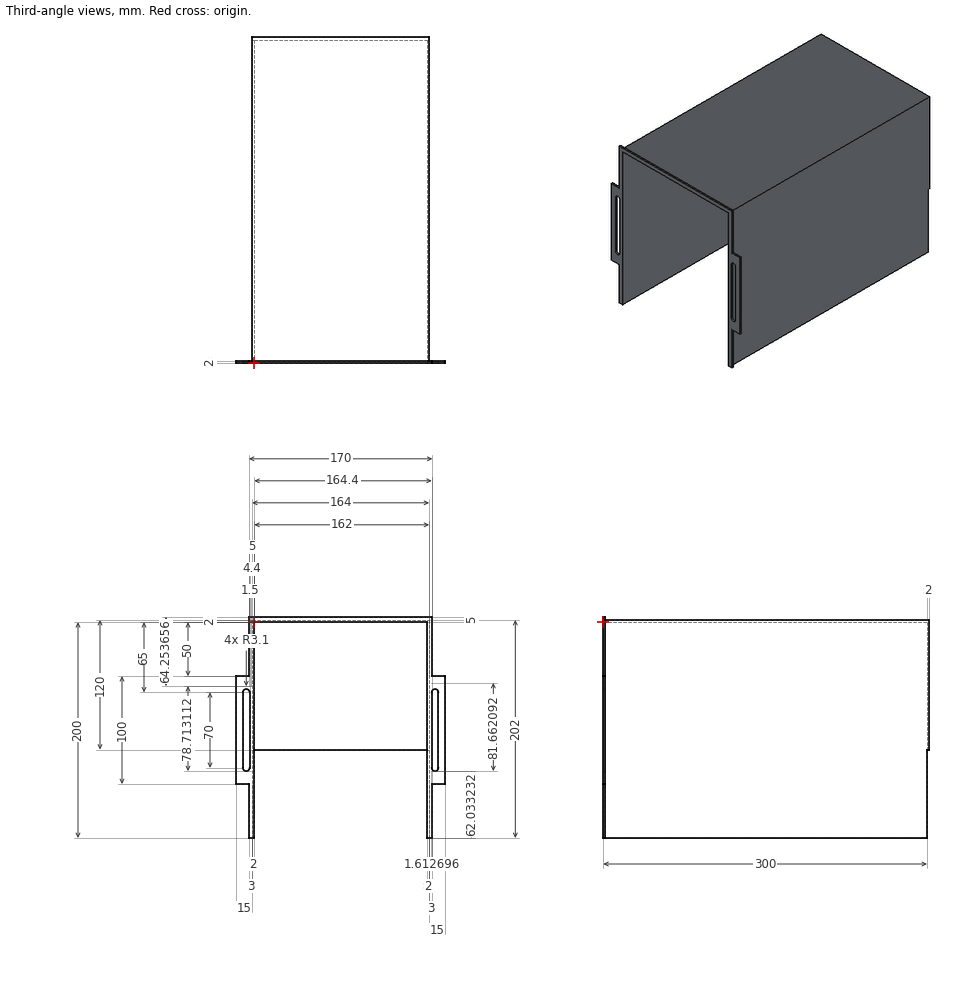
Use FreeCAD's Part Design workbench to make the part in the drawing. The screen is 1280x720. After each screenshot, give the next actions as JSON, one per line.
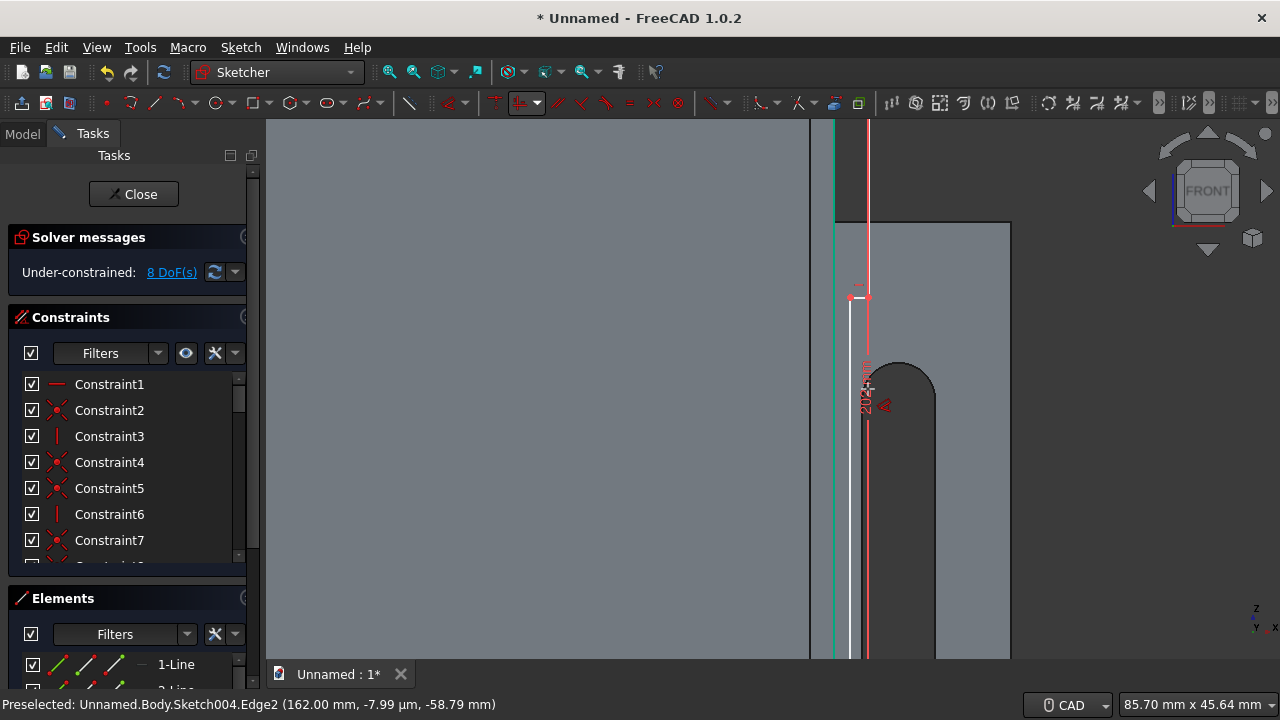
{"action": "scroll", "coordinate": [836, 327], "scroll_direction": "down", "scroll_amount": 10}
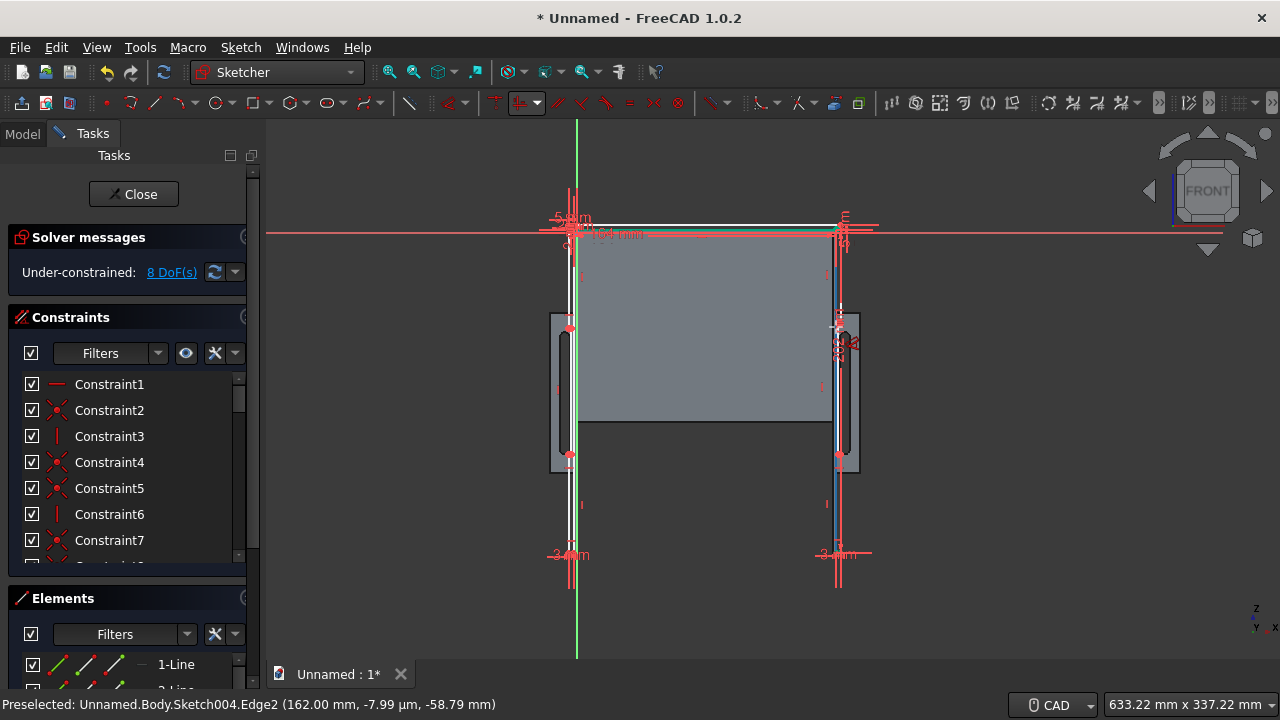
{"action": "scroll", "coordinate": [759, 225], "scroll_direction": "up", "scroll_amount": 6}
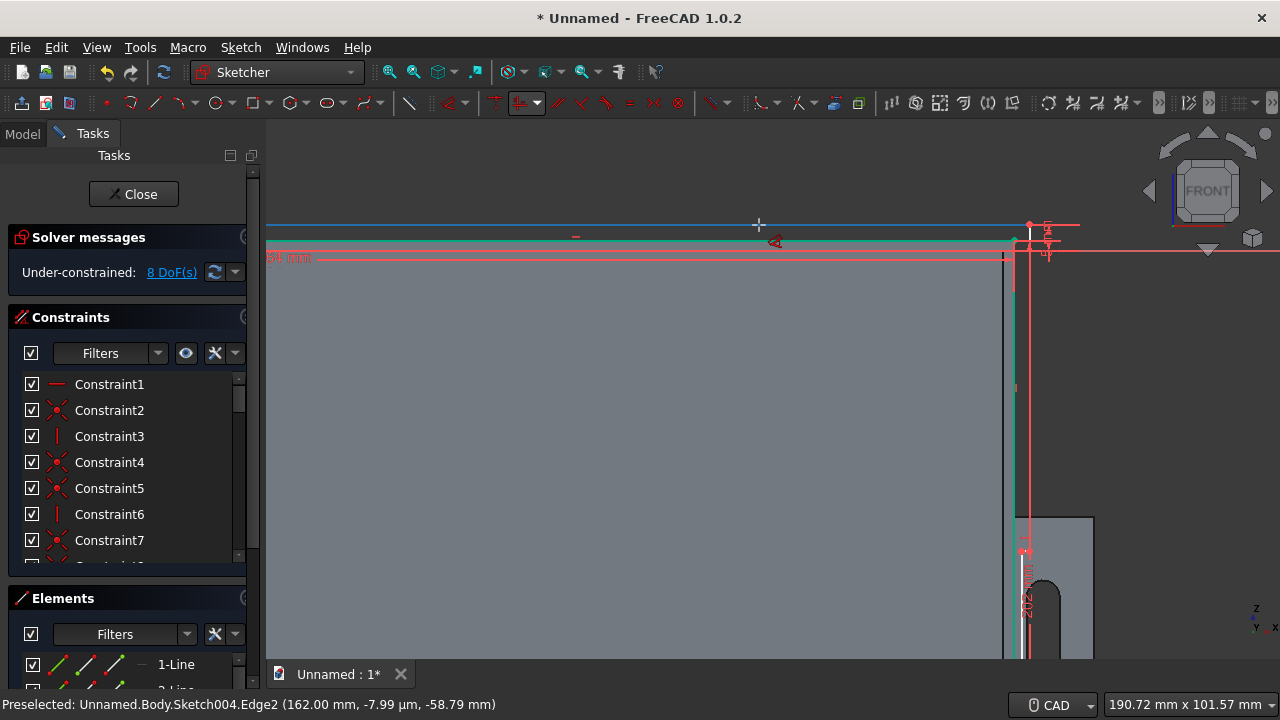
{"action": "left_click", "coordinate": [759, 225]}
{"action": "left_click", "coordinate": [662, 191]}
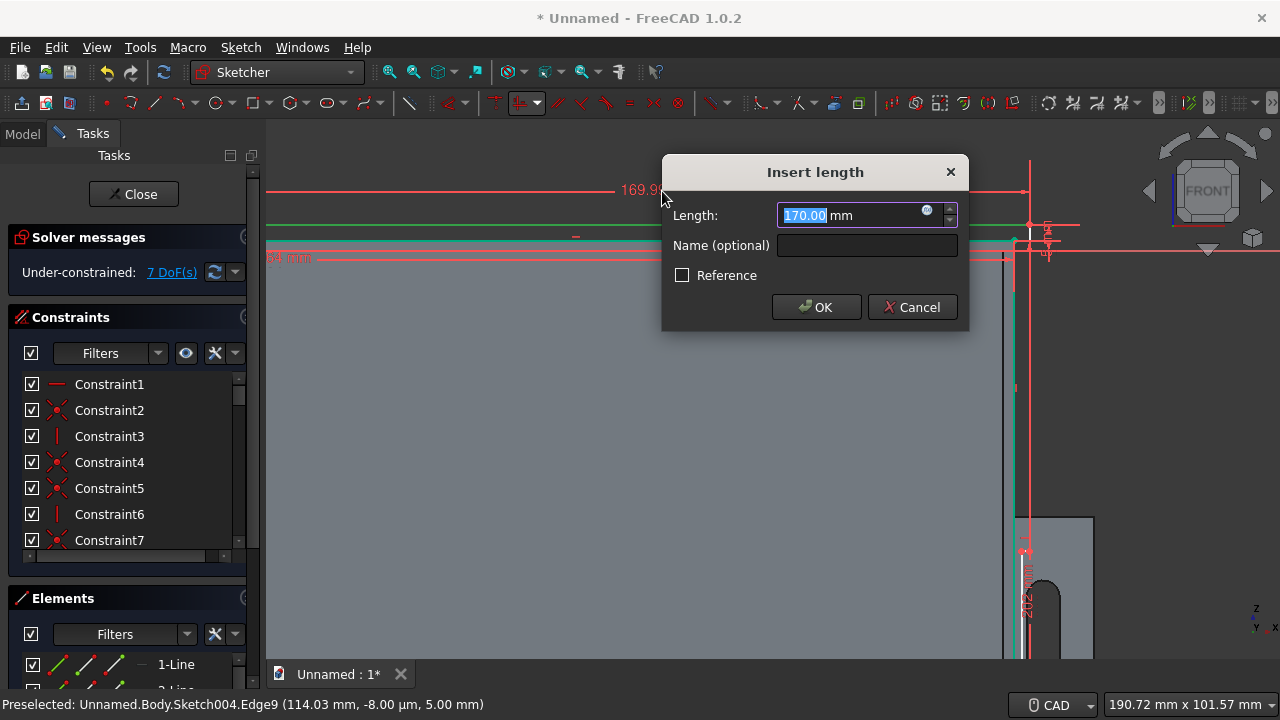
{"action": "type", "text": "170"}
{"action": "key", "text": "Return"}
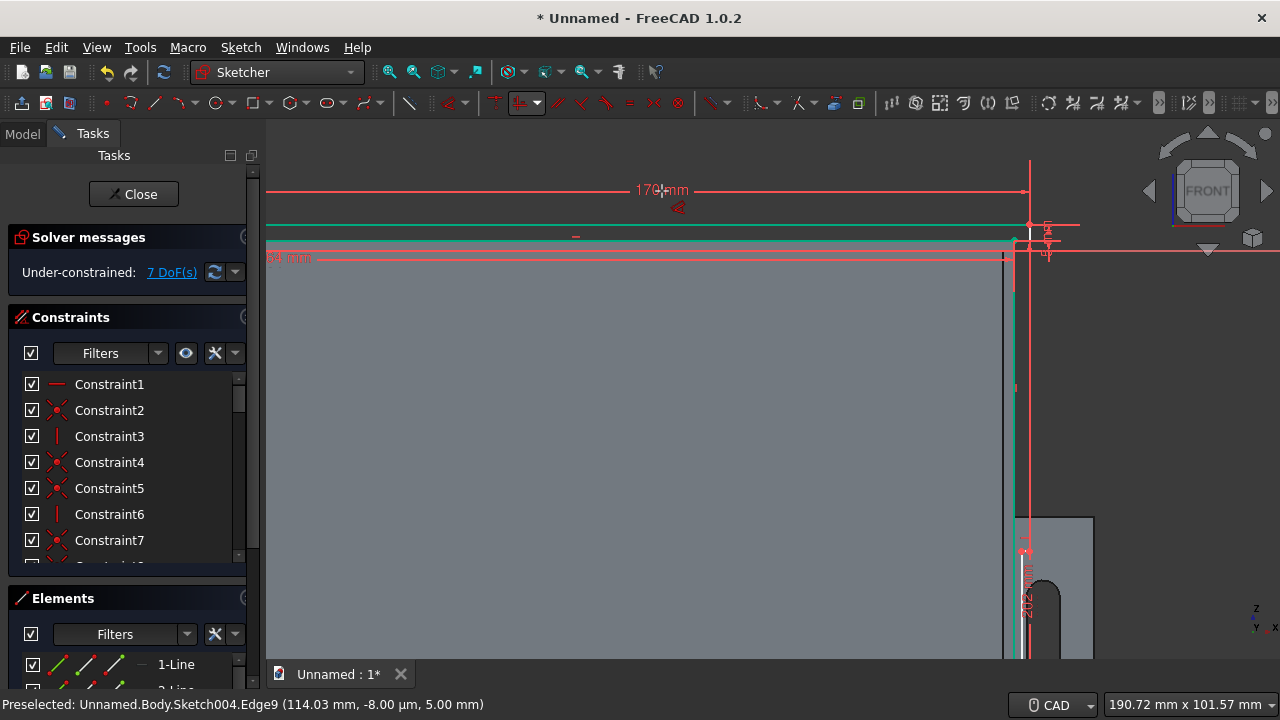
{"action": "scroll", "coordinate": [759, 225], "scroll_direction": "down", "scroll_amount": 6}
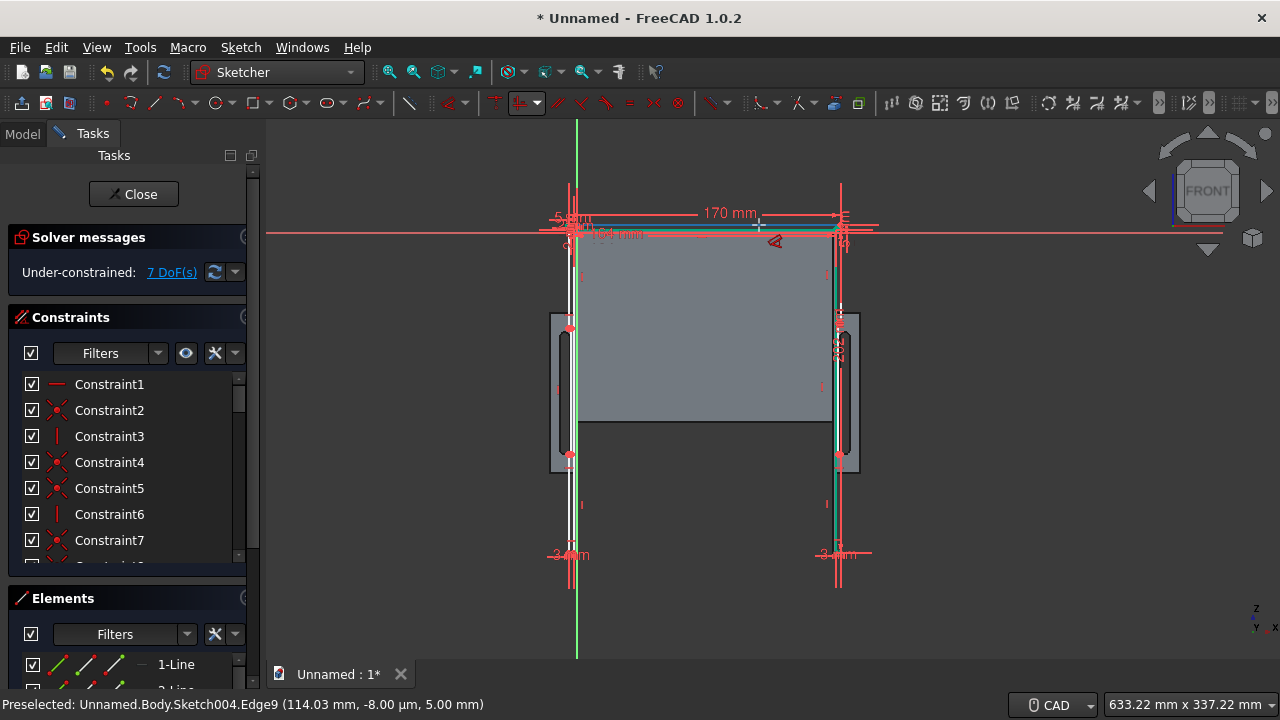
{"action": "scroll", "coordinate": [570, 328], "scroll_direction": "up", "scroll_amount": 15}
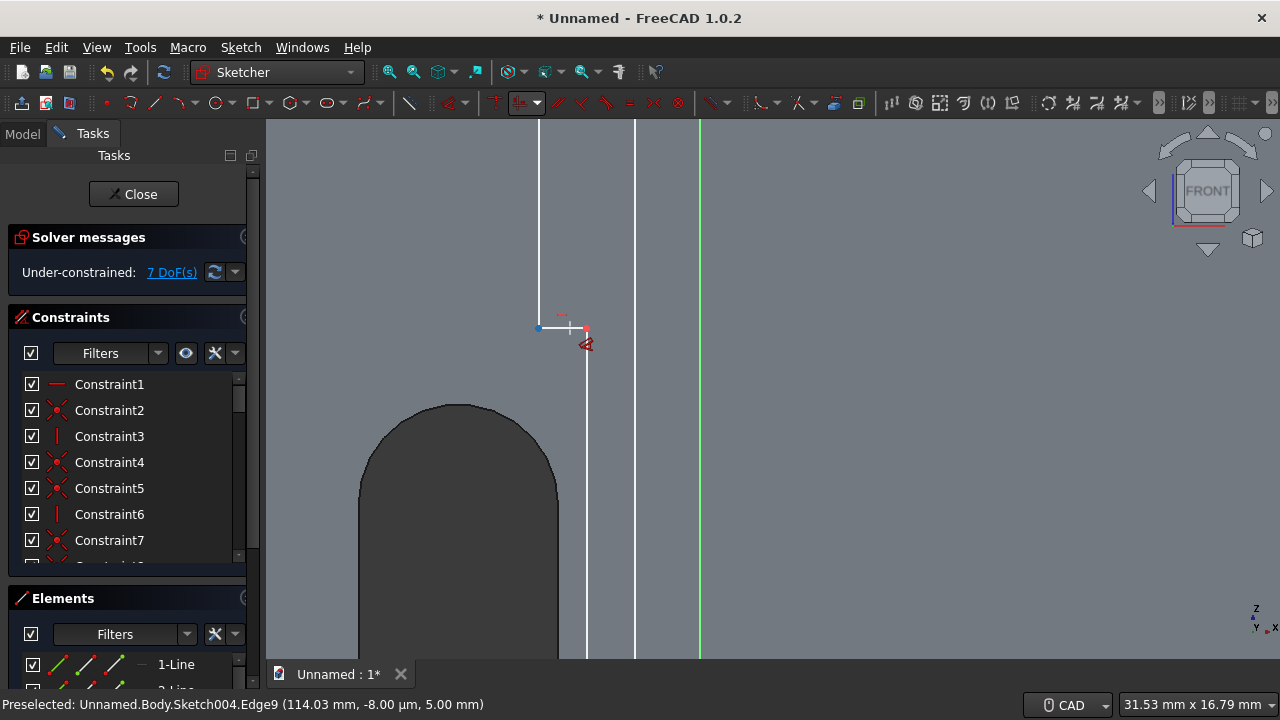
{"action": "left_click", "coordinate": [563, 328]}
{"action": "left_click", "coordinate": [563, 294]}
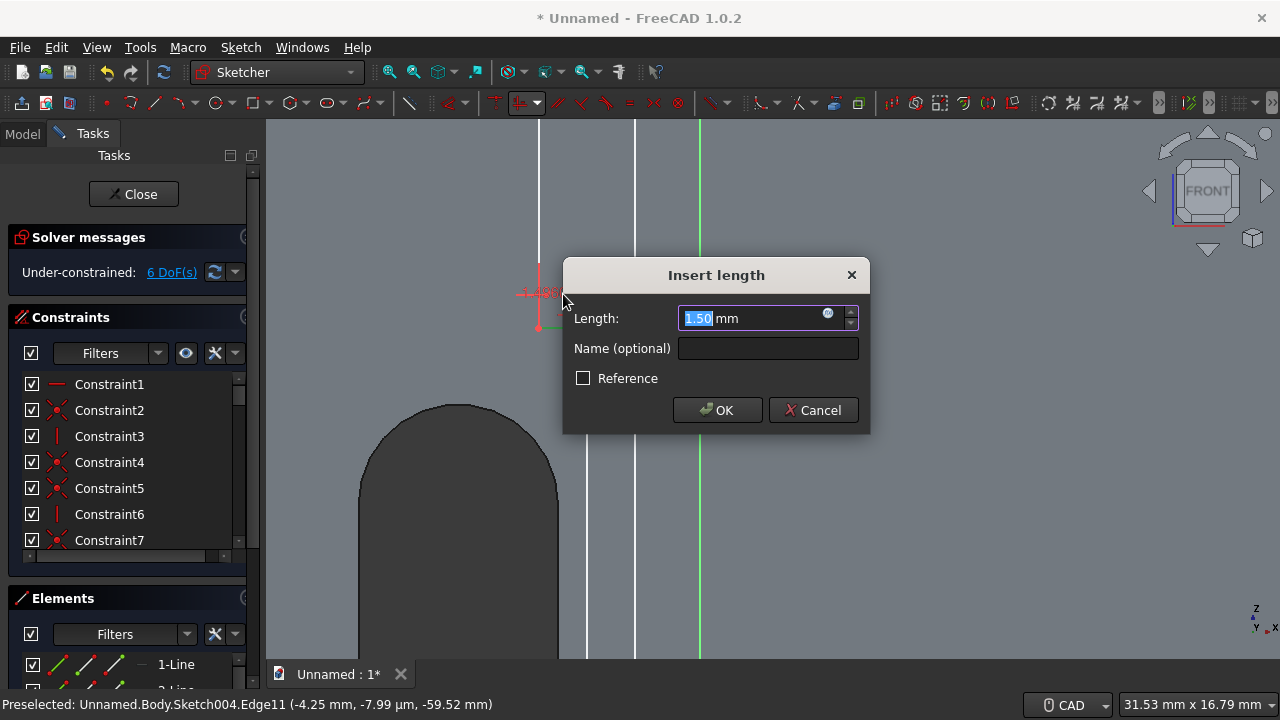
{"action": "type", "text": "1.5"}
{"action": "key", "text": "Return"}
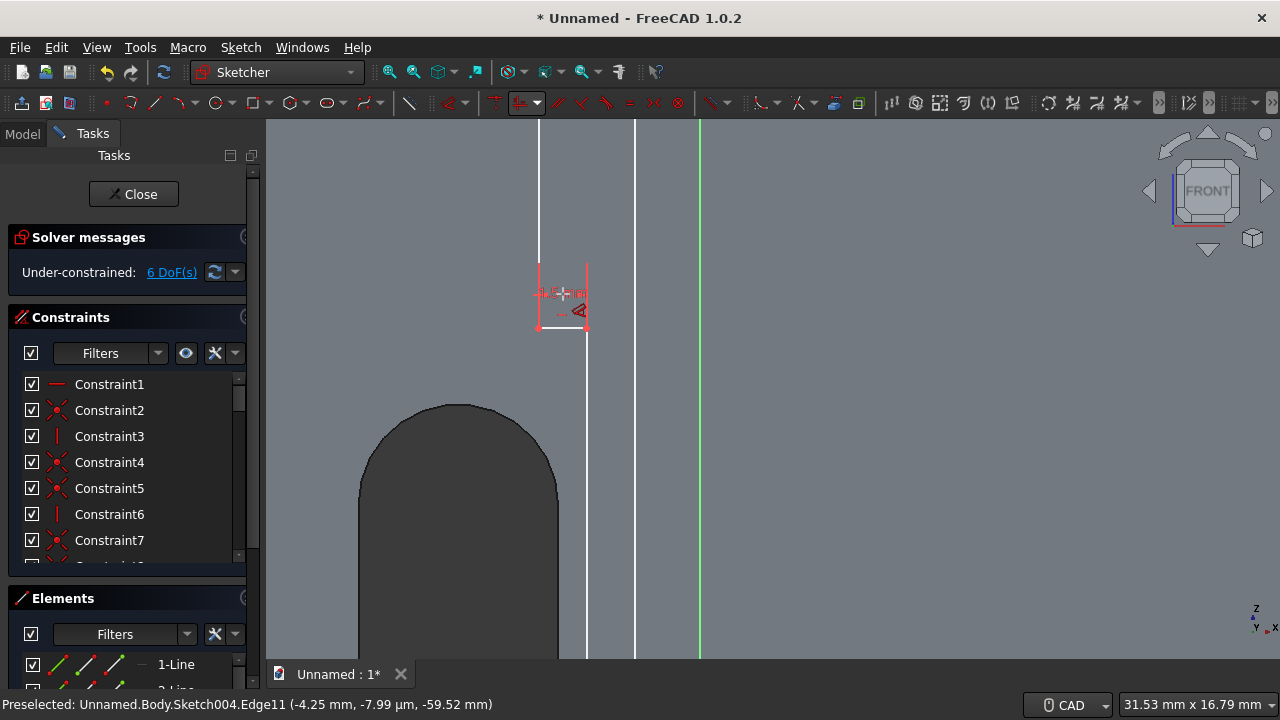
{"action": "scroll", "coordinate": [570, 328], "scroll_direction": "down", "scroll_amount": 15}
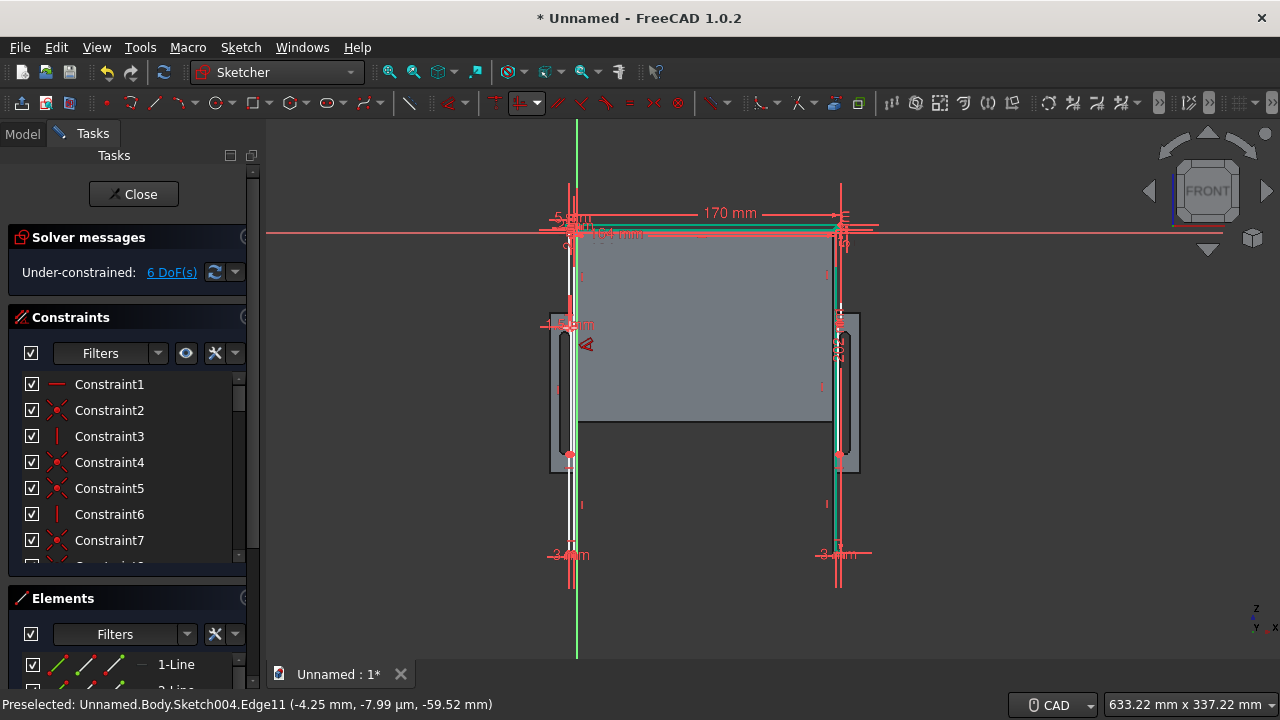
{"action": "scroll", "coordinate": [574, 327], "scroll_direction": "up", "scroll_amount": 9}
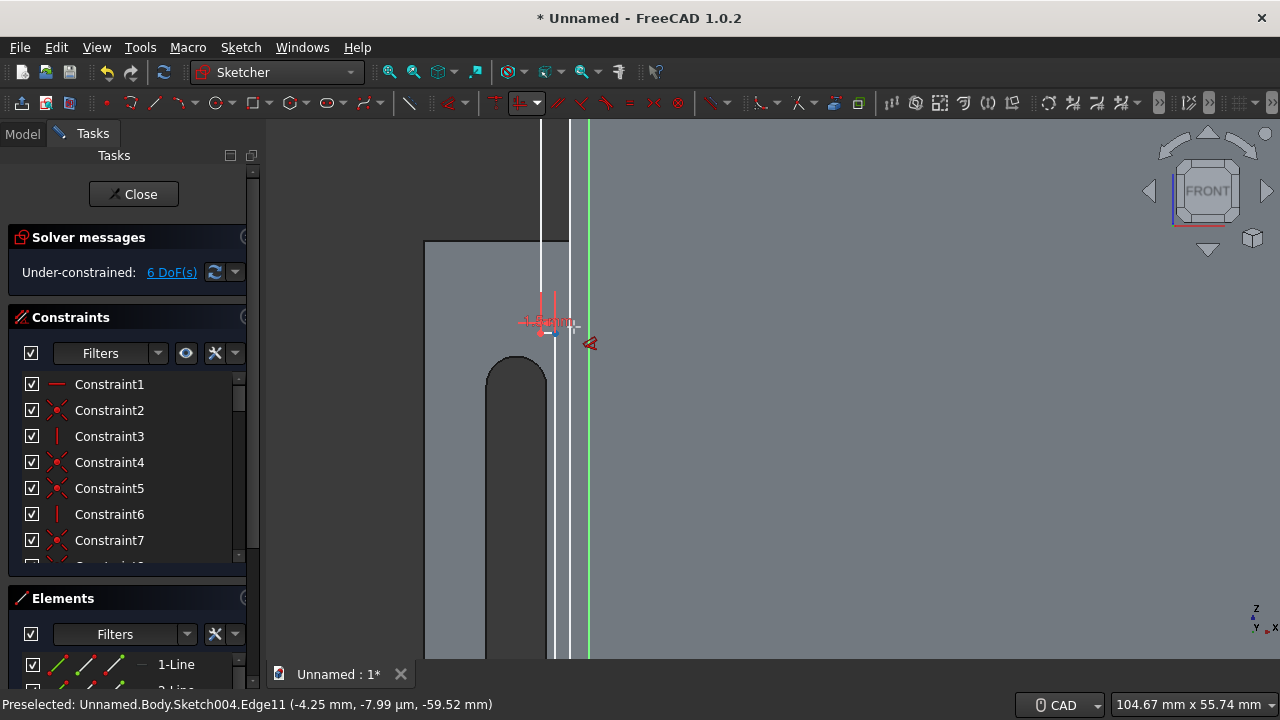
{"action": "left_click", "coordinate": [570, 325]}
{"action": "left_click", "coordinate": [536, 389]}